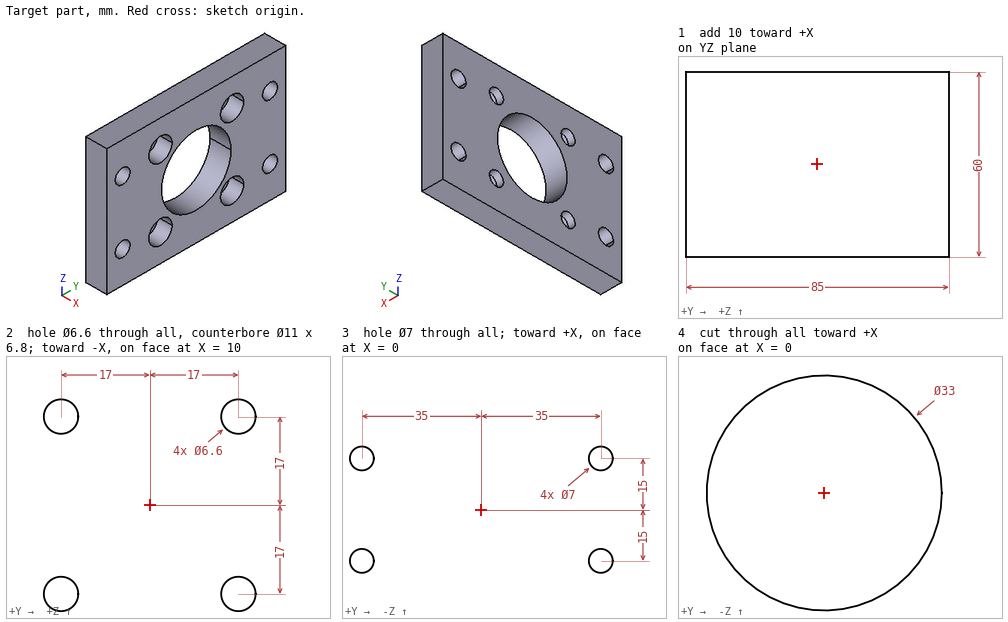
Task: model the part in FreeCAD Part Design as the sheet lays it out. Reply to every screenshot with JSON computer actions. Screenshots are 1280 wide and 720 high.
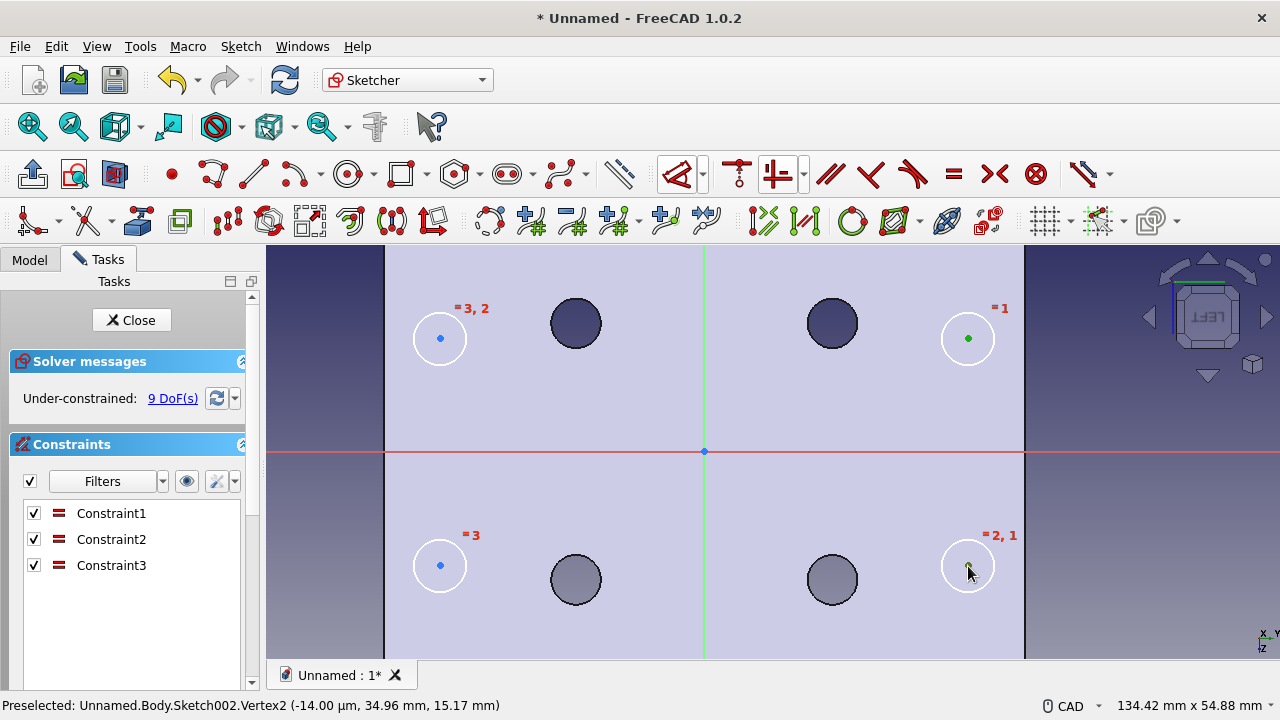
{"action": "left_click", "coordinate": [804, 174]}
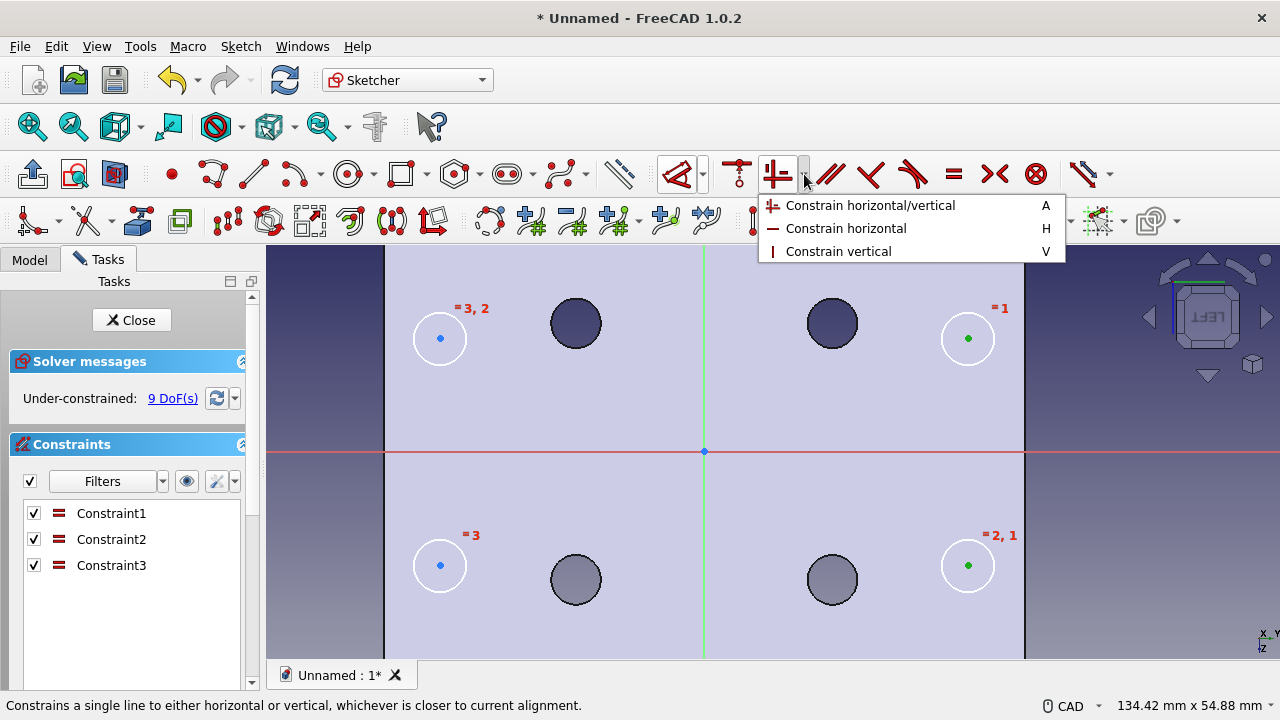
{"action": "left_click", "coordinate": [912, 252]}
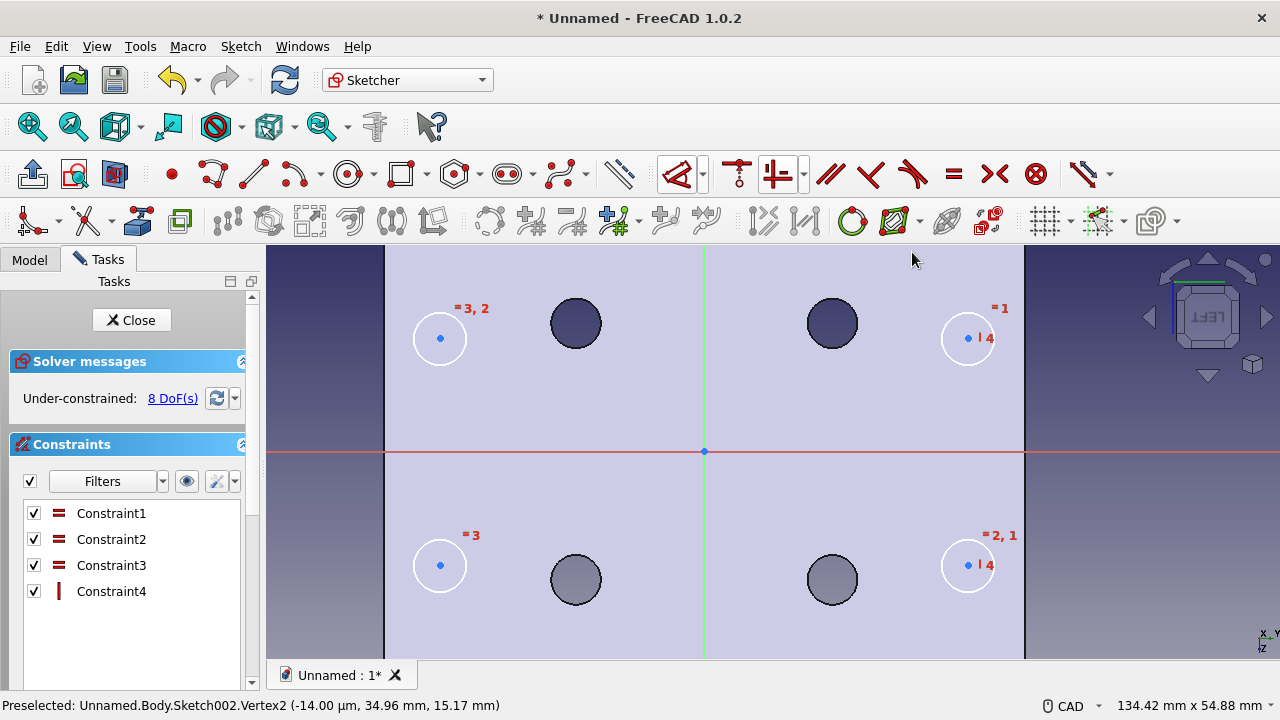
{"action": "left_click", "coordinate": [968, 339]}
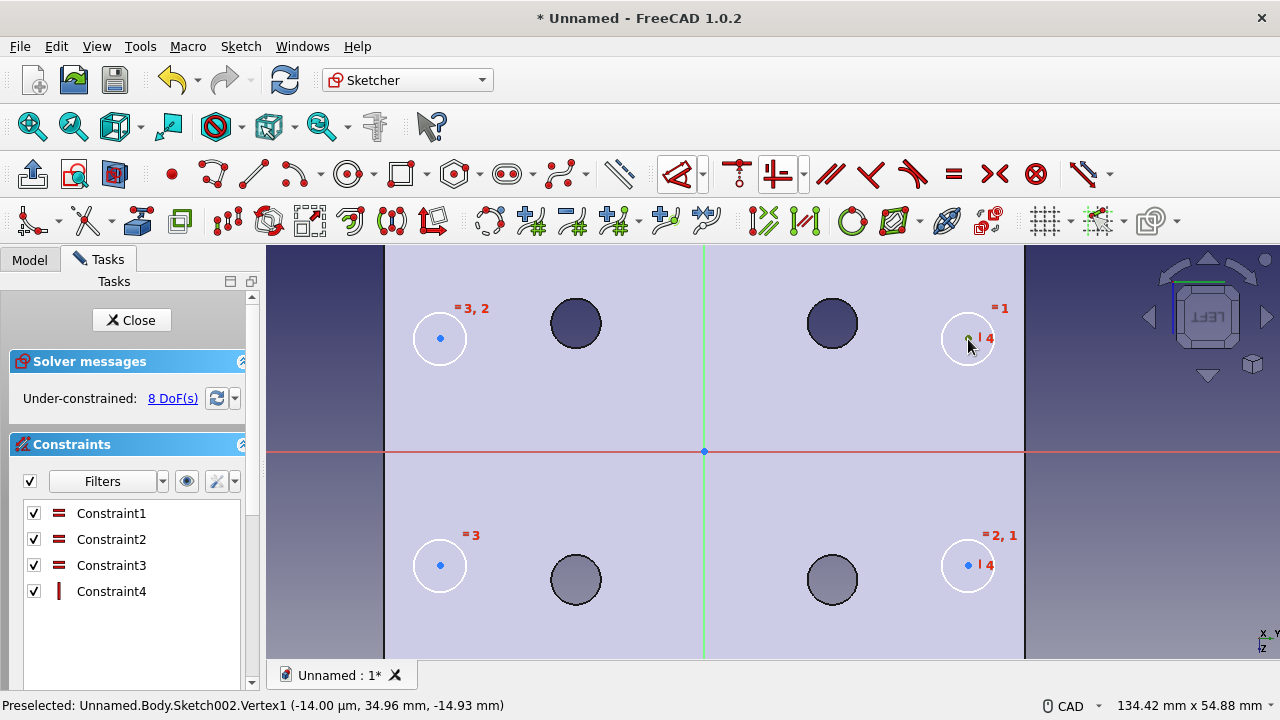
{"action": "left_click", "coordinate": [440, 339]}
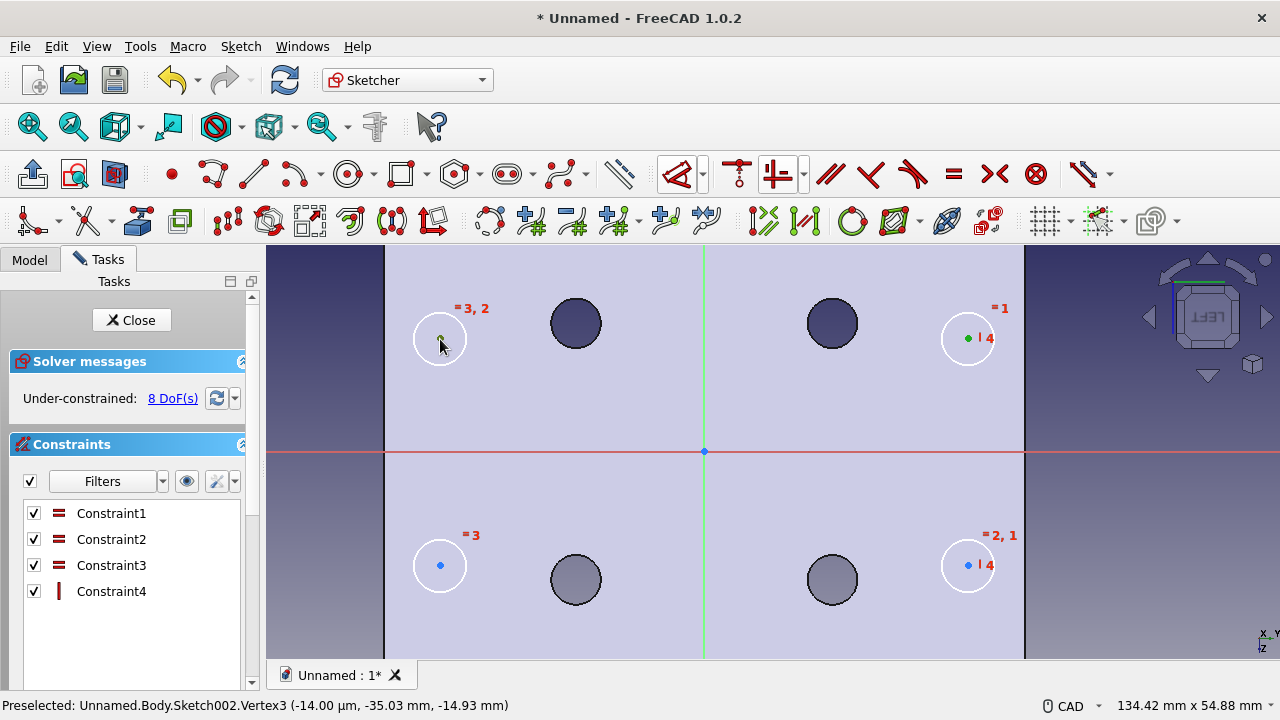
{"action": "key", "text": "h"}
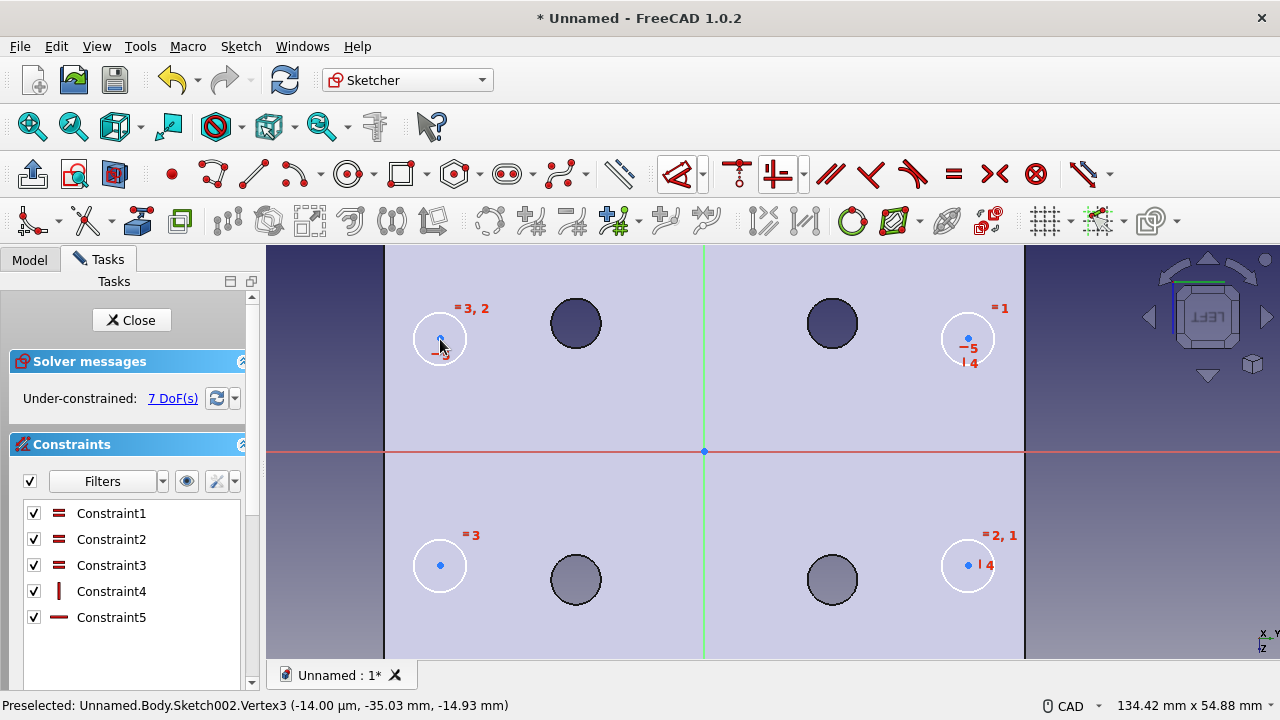
{"action": "left_click", "coordinate": [440, 339]}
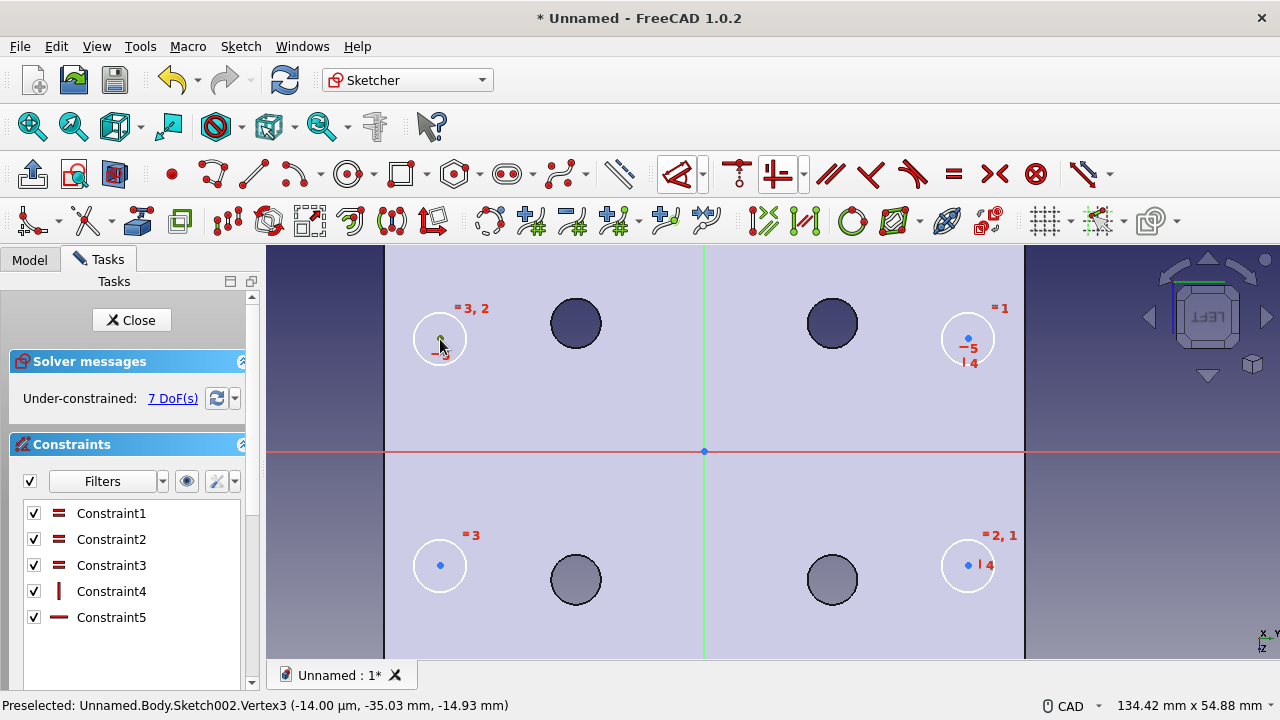
{"action": "left_click", "coordinate": [440, 566]}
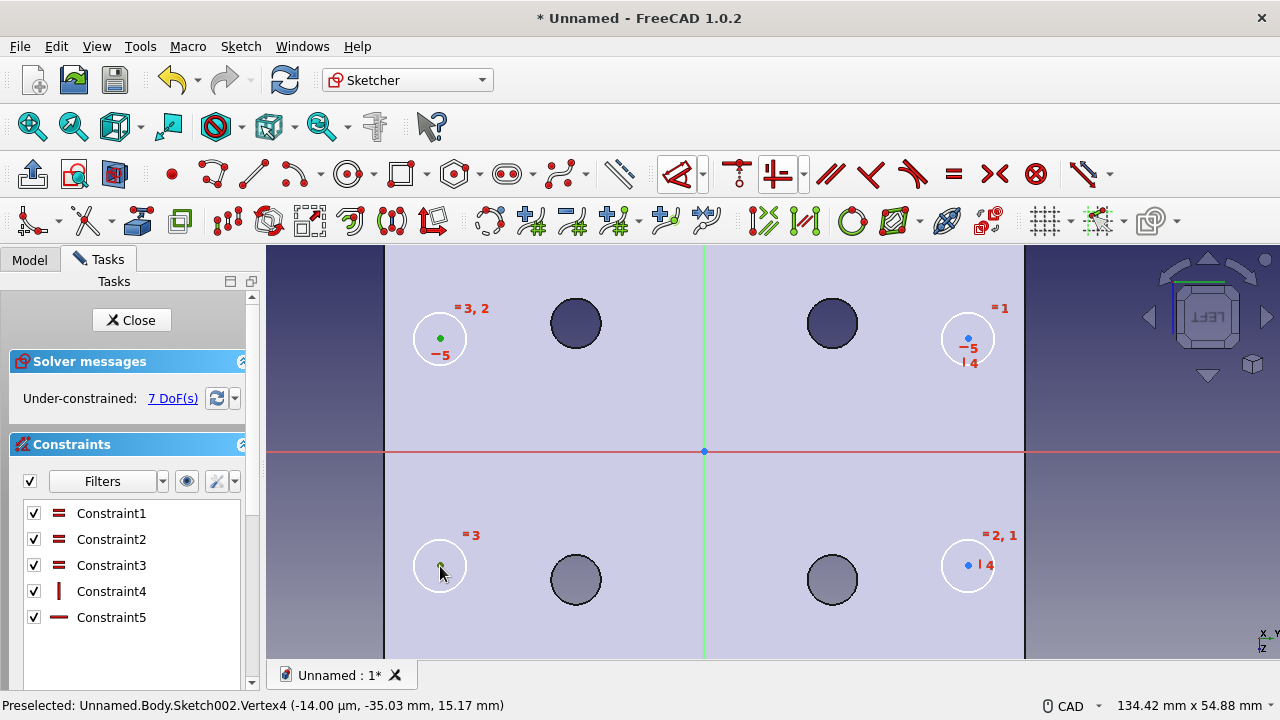
{"action": "key", "text": "v"}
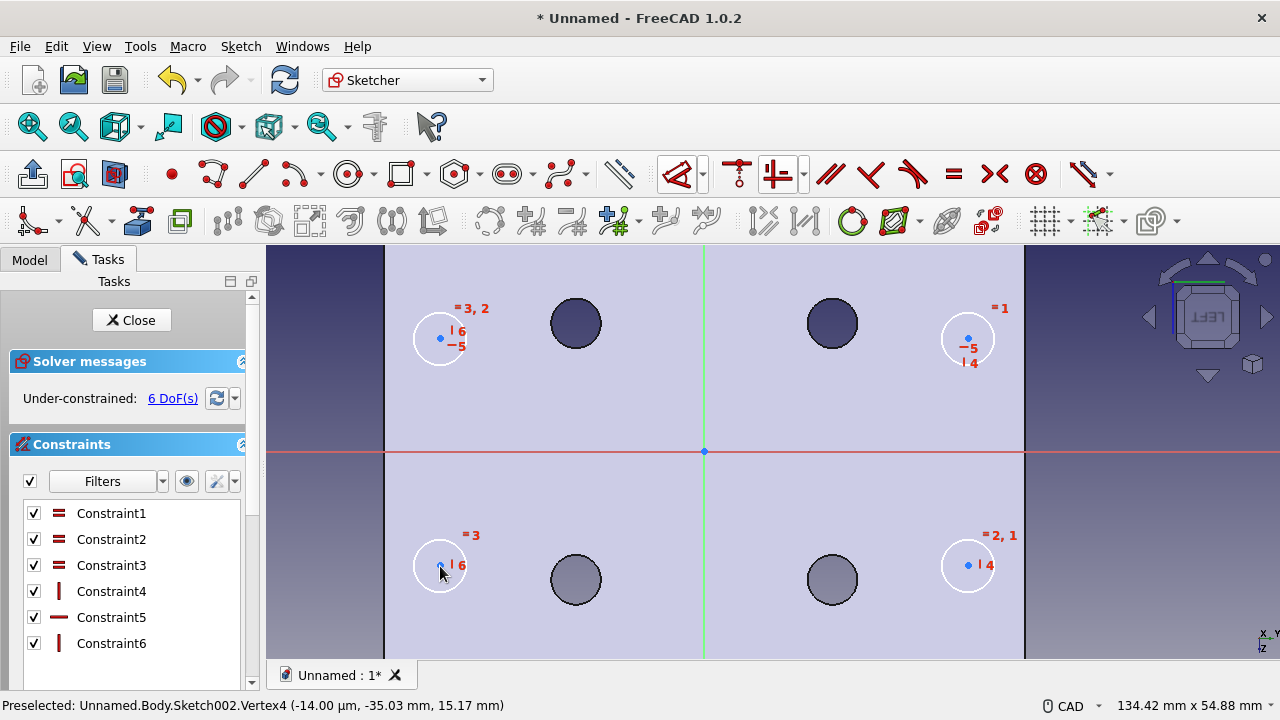
{"action": "left_click", "coordinate": [968, 566]}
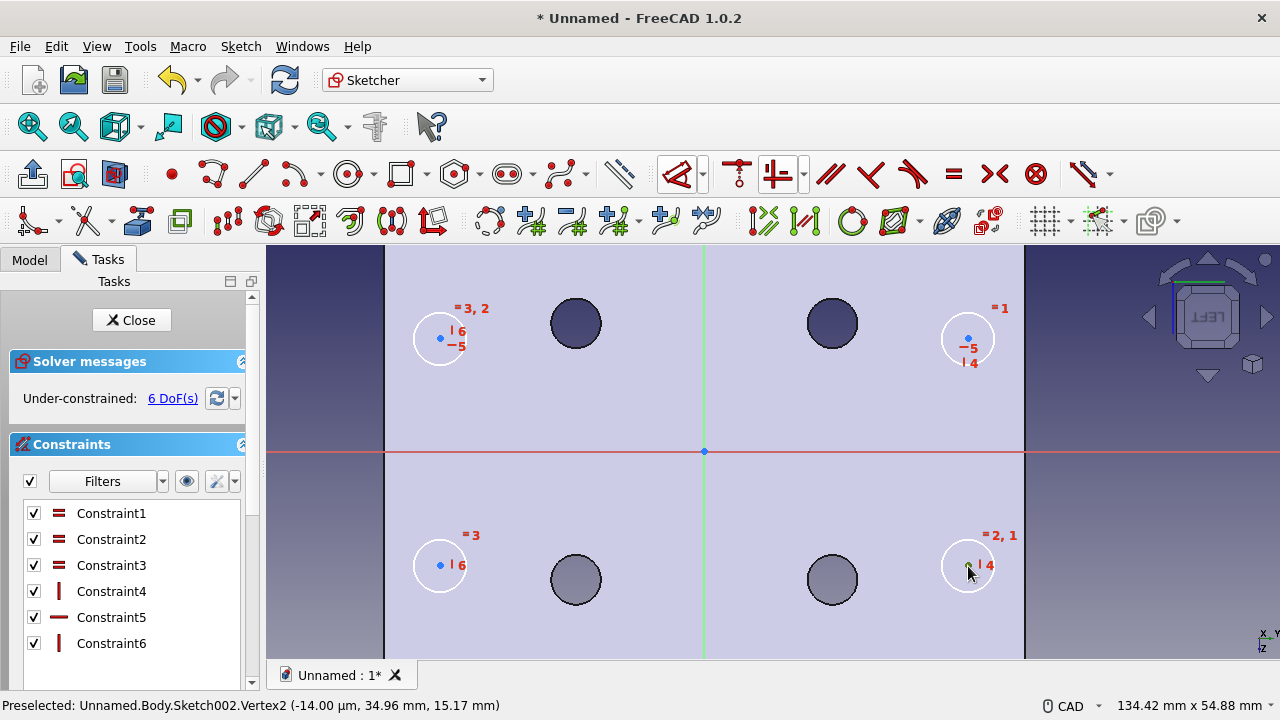
{"action": "left_click", "coordinate": [440, 566]}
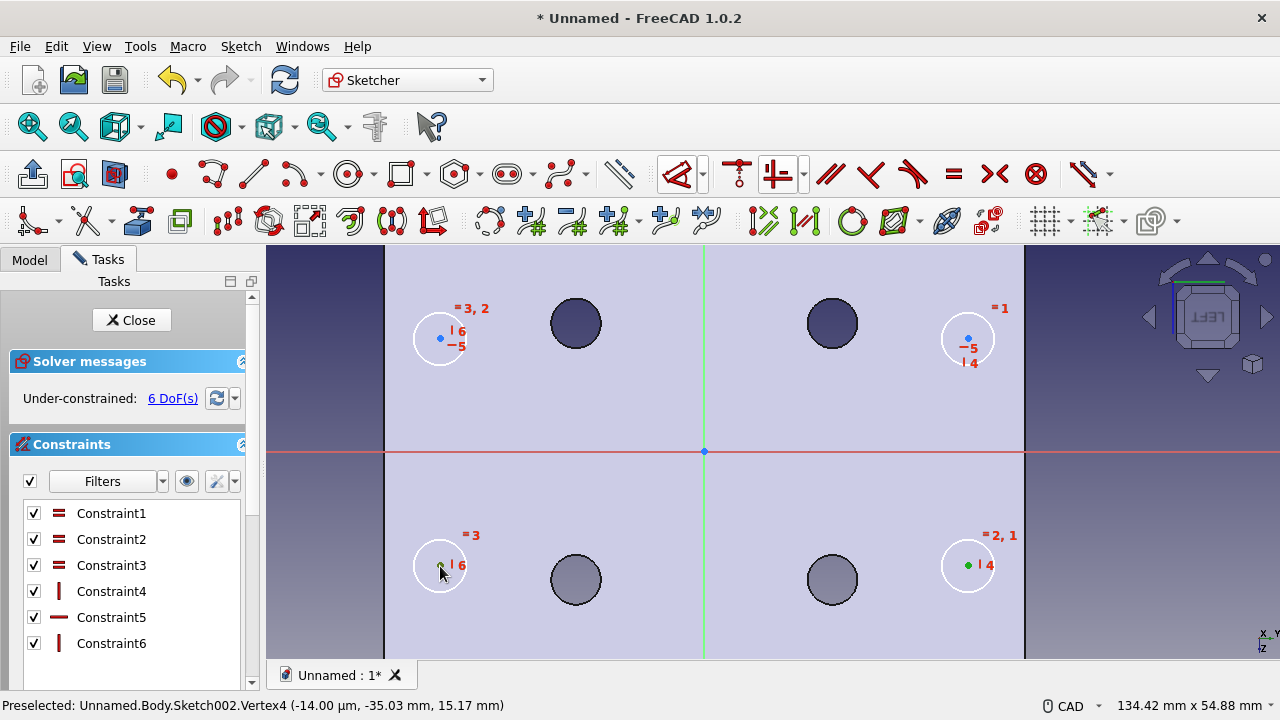
{"action": "left_click", "coordinate": [804, 174]}